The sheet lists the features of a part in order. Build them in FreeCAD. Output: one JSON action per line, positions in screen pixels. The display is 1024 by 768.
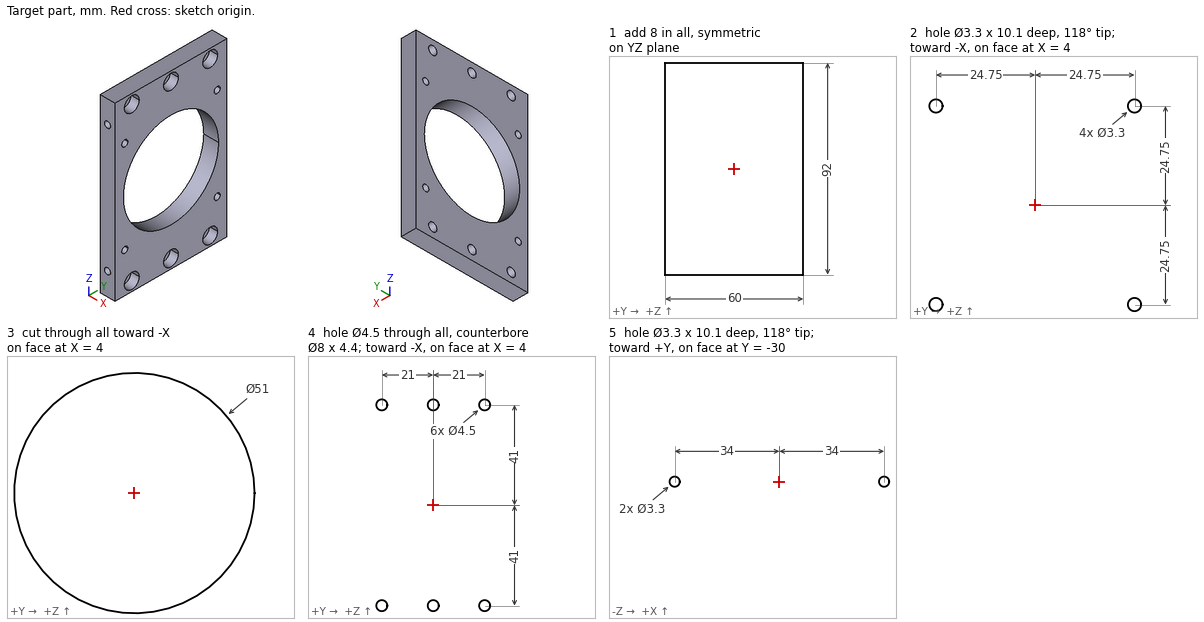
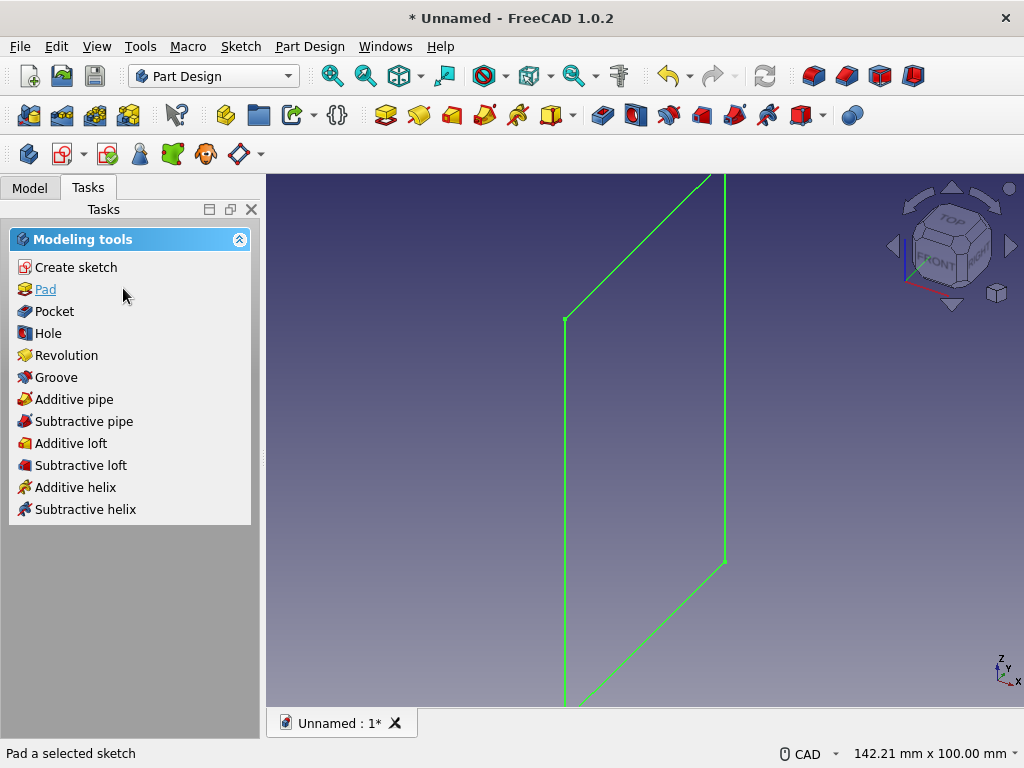
{"action": "left_click", "coordinate": [386, 116]}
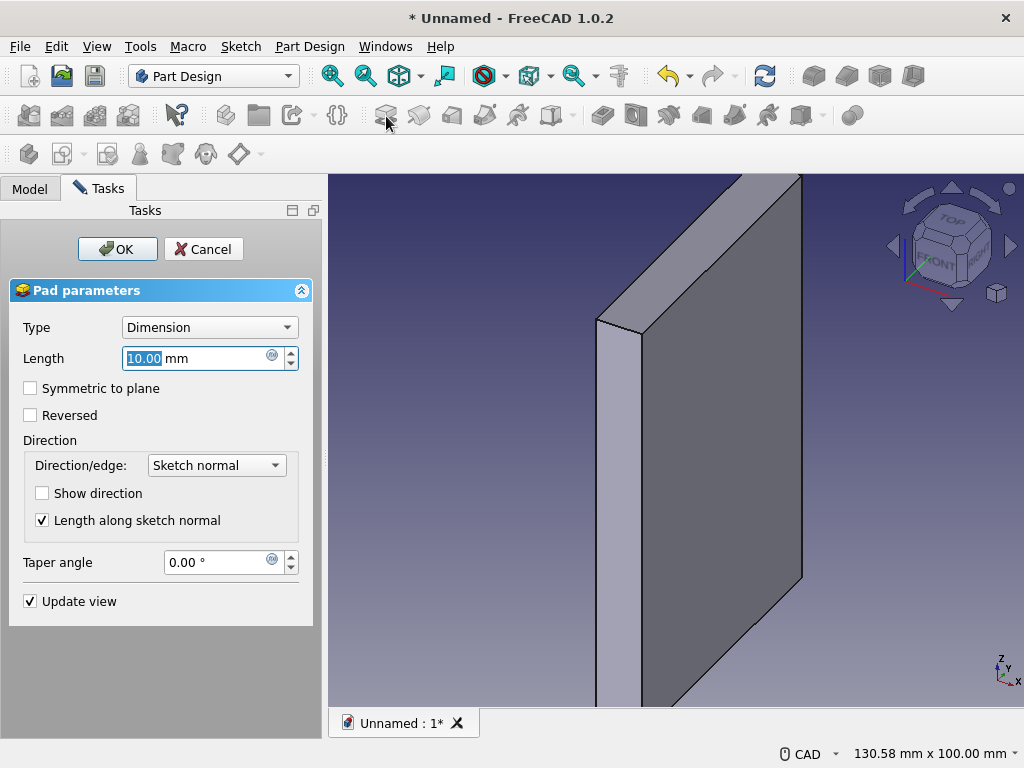
{"action": "type", "text": "8"}
{"action": "key", "text": "Tab"}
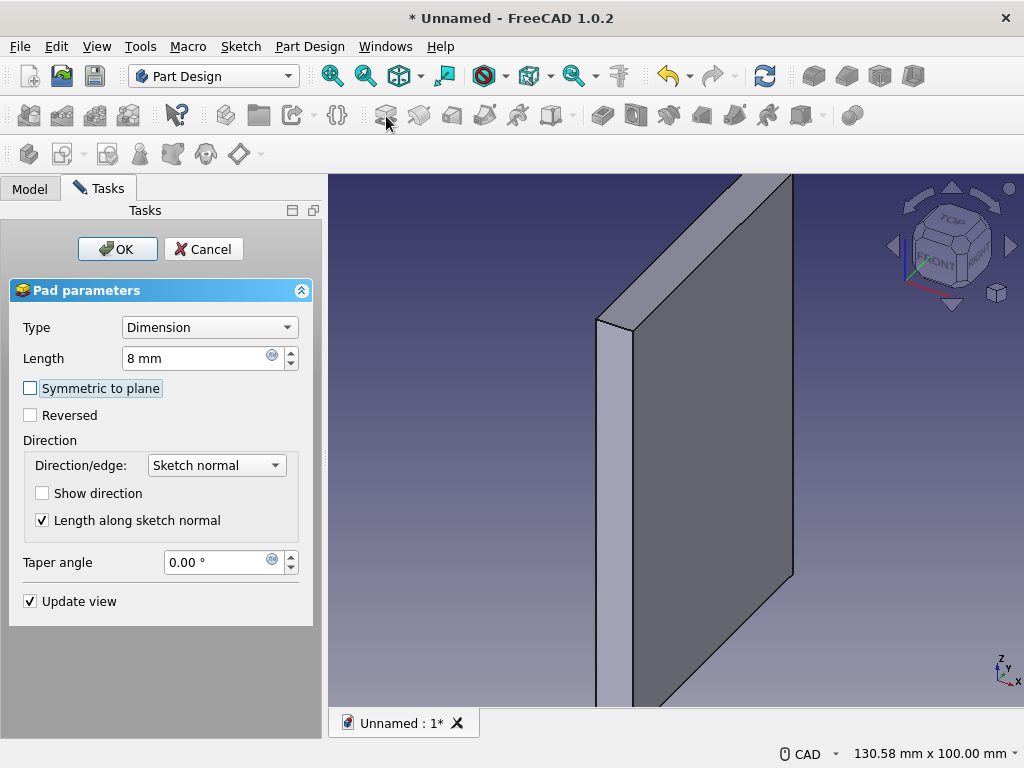
{"action": "left_click", "coordinate": [31, 388]}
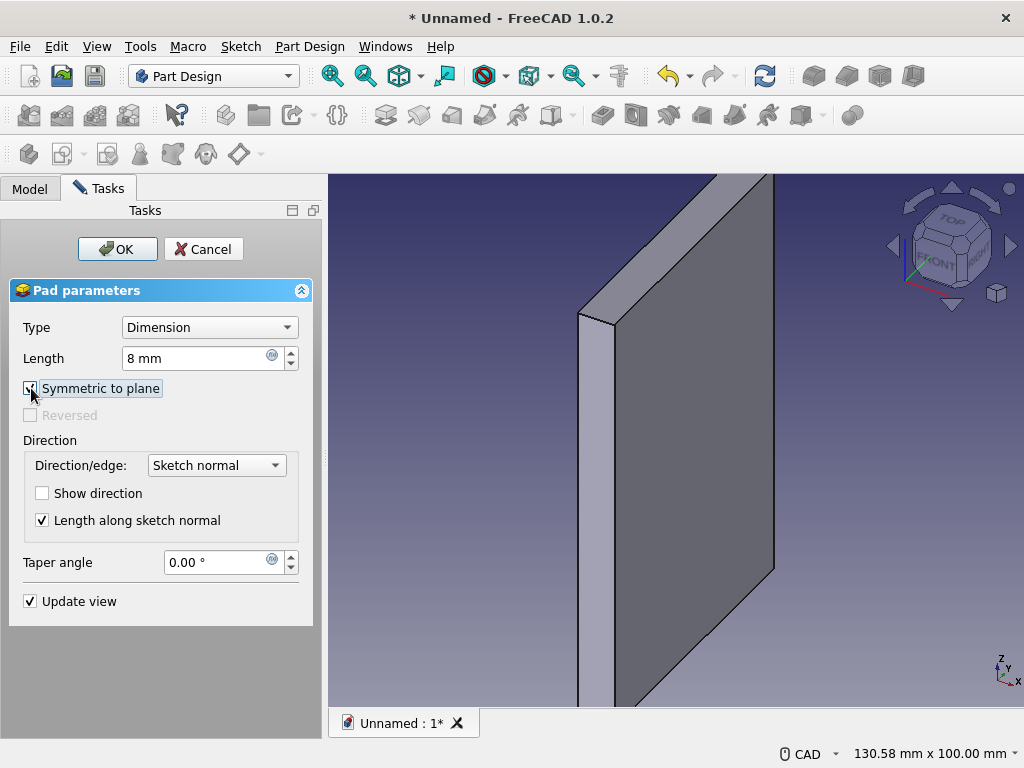
{"action": "left_click", "coordinate": [118, 249]}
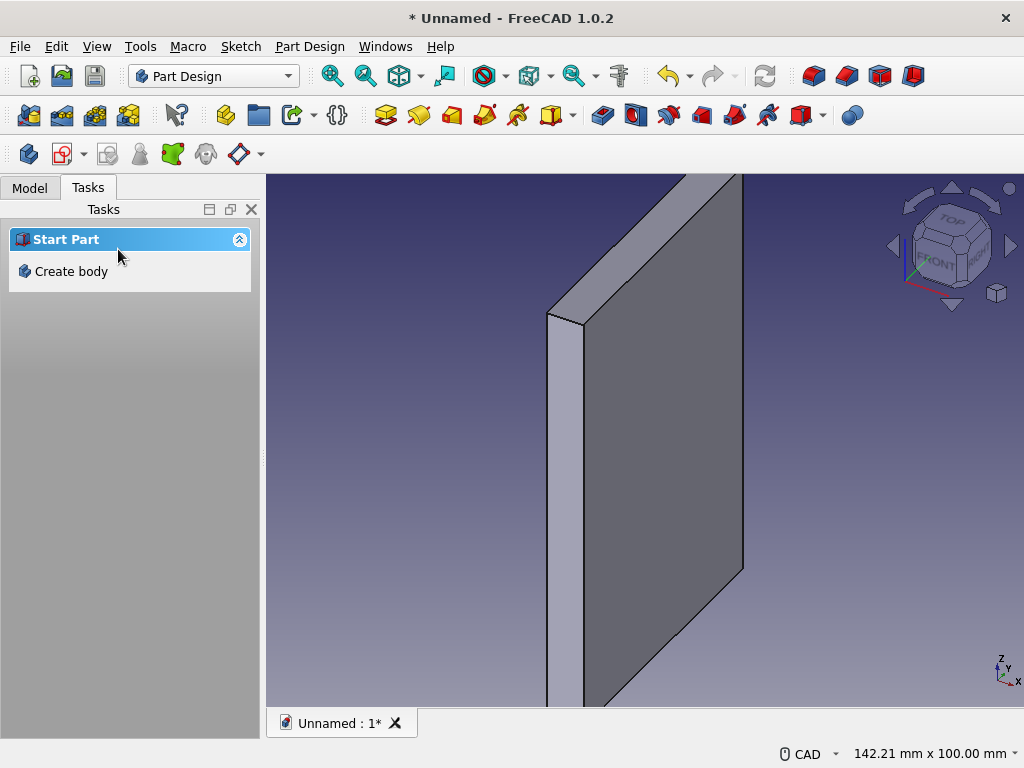
{"action": "left_click", "coordinate": [333, 76]}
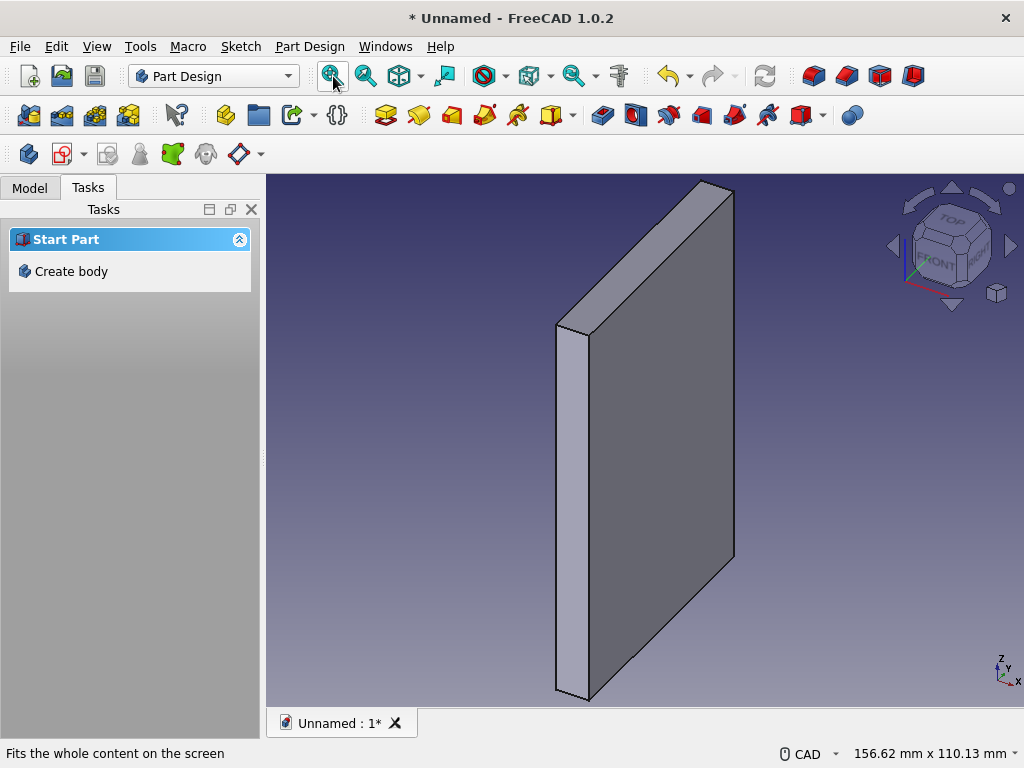
{"action": "left_click", "coordinate": [662, 497]}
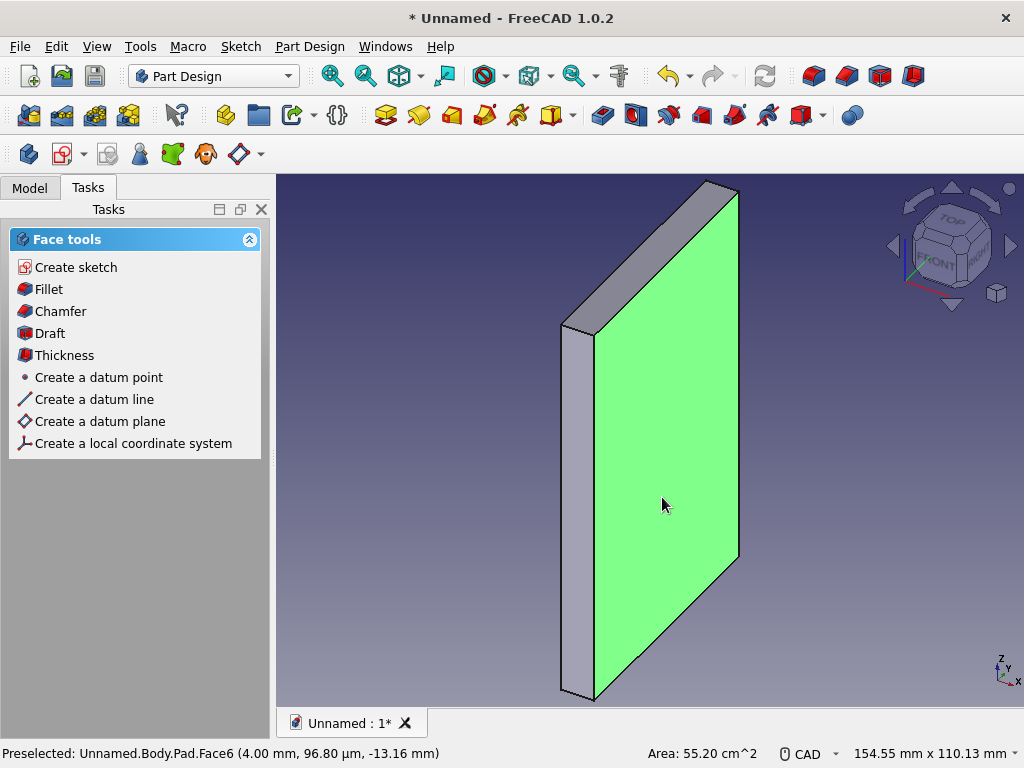
{"action": "left_click", "coordinate": [62, 154]}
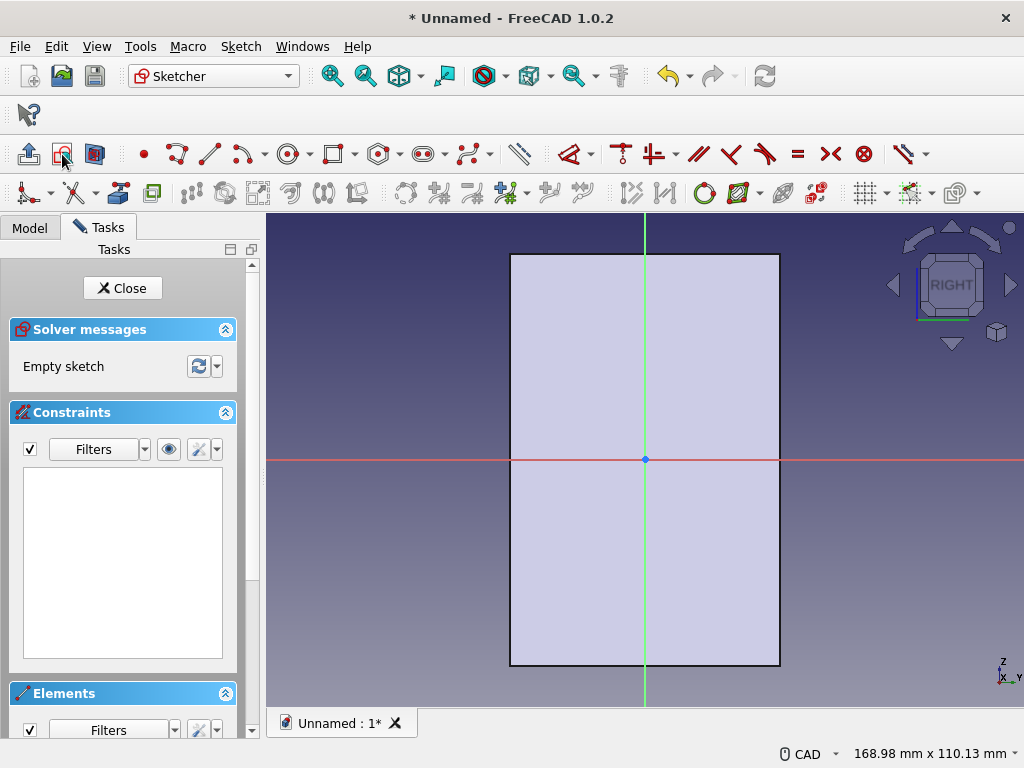
{"action": "left_click", "coordinate": [288, 154]}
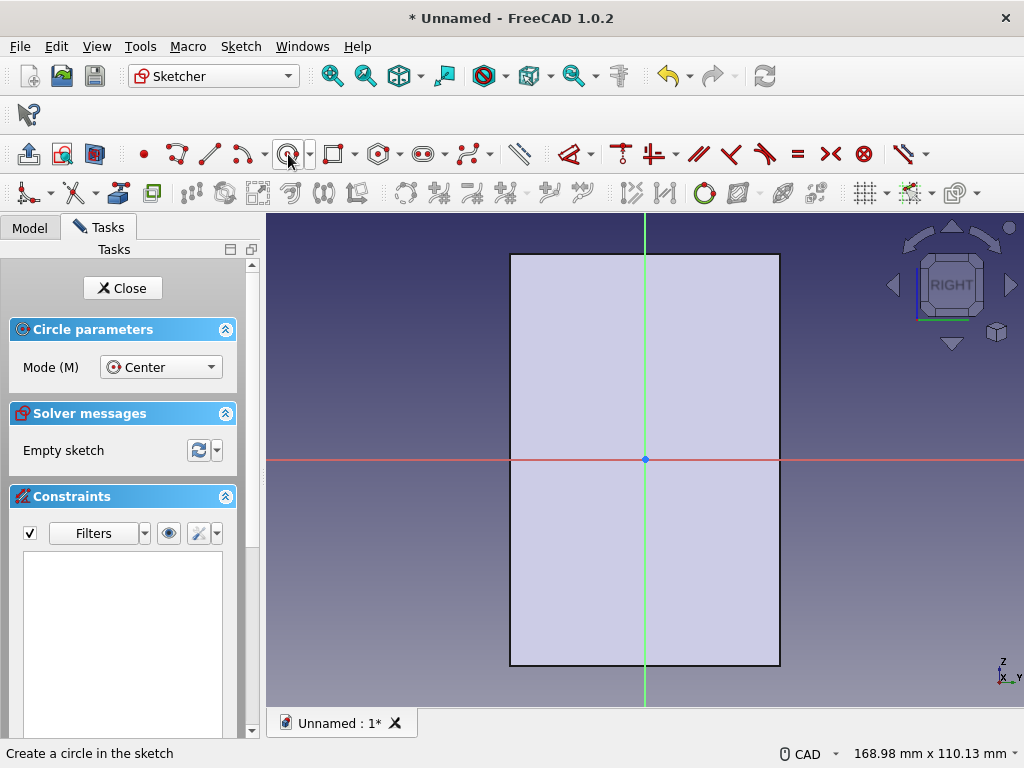
{"action": "scroll", "coordinate": [756, 349], "scroll_direction": "up", "scroll_amount": 6}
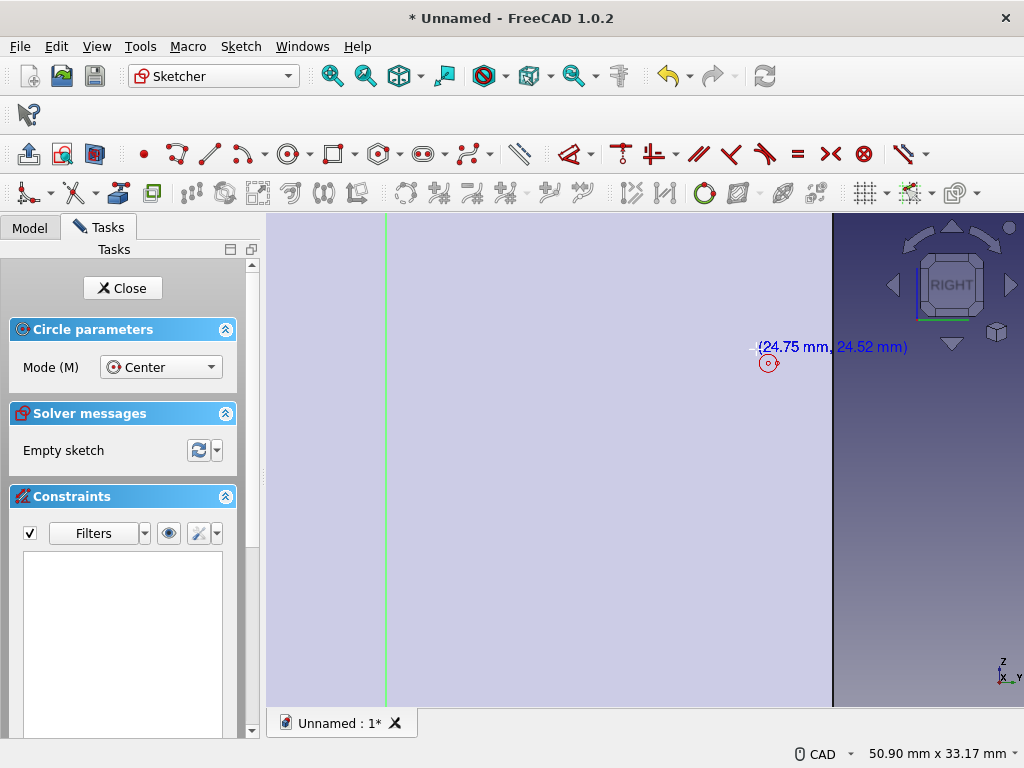
{"action": "left_click", "coordinate": [755, 348]}
{"action": "left_click", "coordinate": [772, 331]}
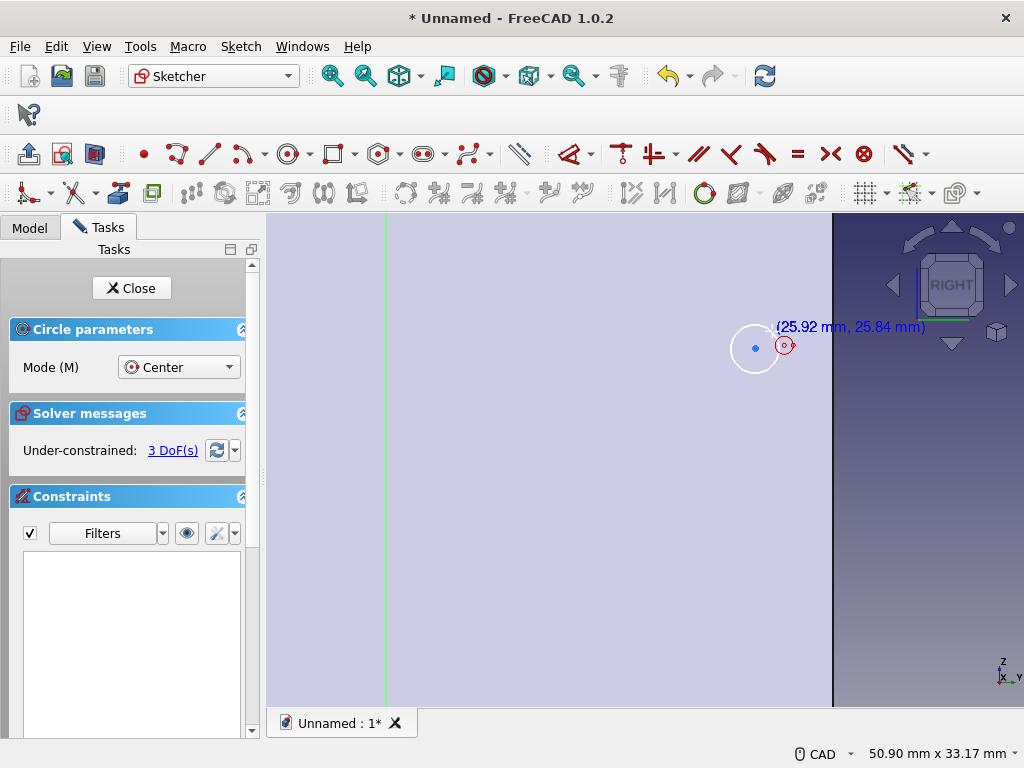
{"action": "scroll", "coordinate": [687, 310], "scroll_direction": "down", "scroll_amount": 5}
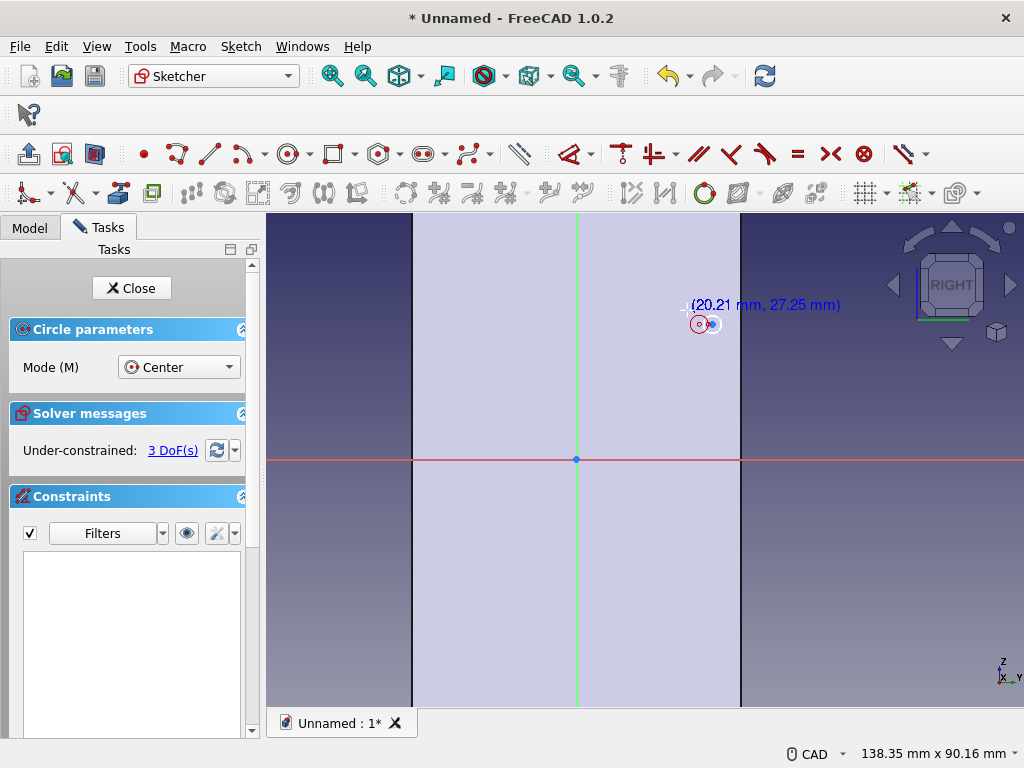
{"action": "scroll", "coordinate": [712, 595], "scroll_direction": "up", "scroll_amount": 5}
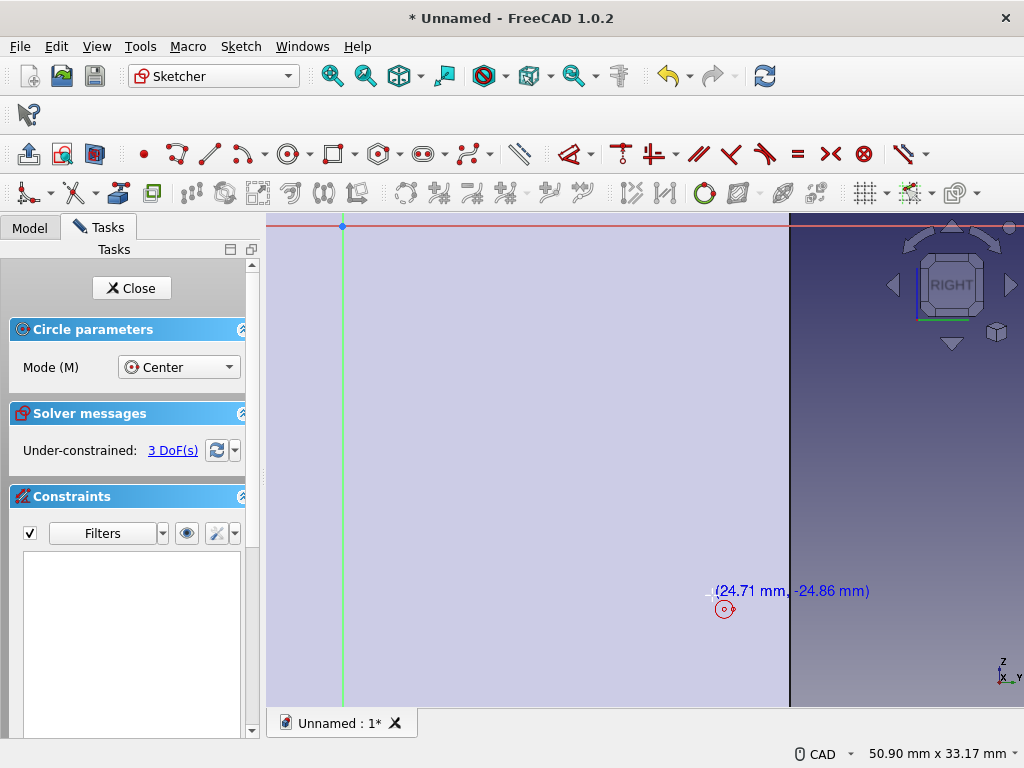
{"action": "left_click", "coordinate": [712, 595]}
{"action": "left_click", "coordinate": [729, 577]}